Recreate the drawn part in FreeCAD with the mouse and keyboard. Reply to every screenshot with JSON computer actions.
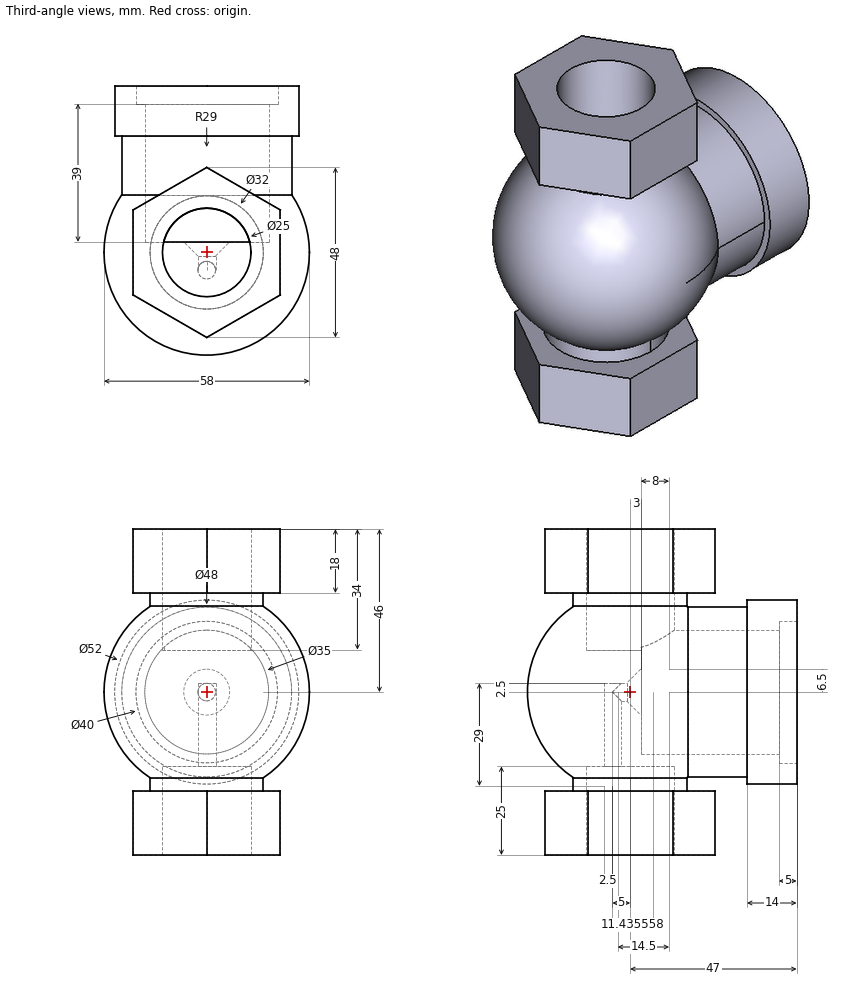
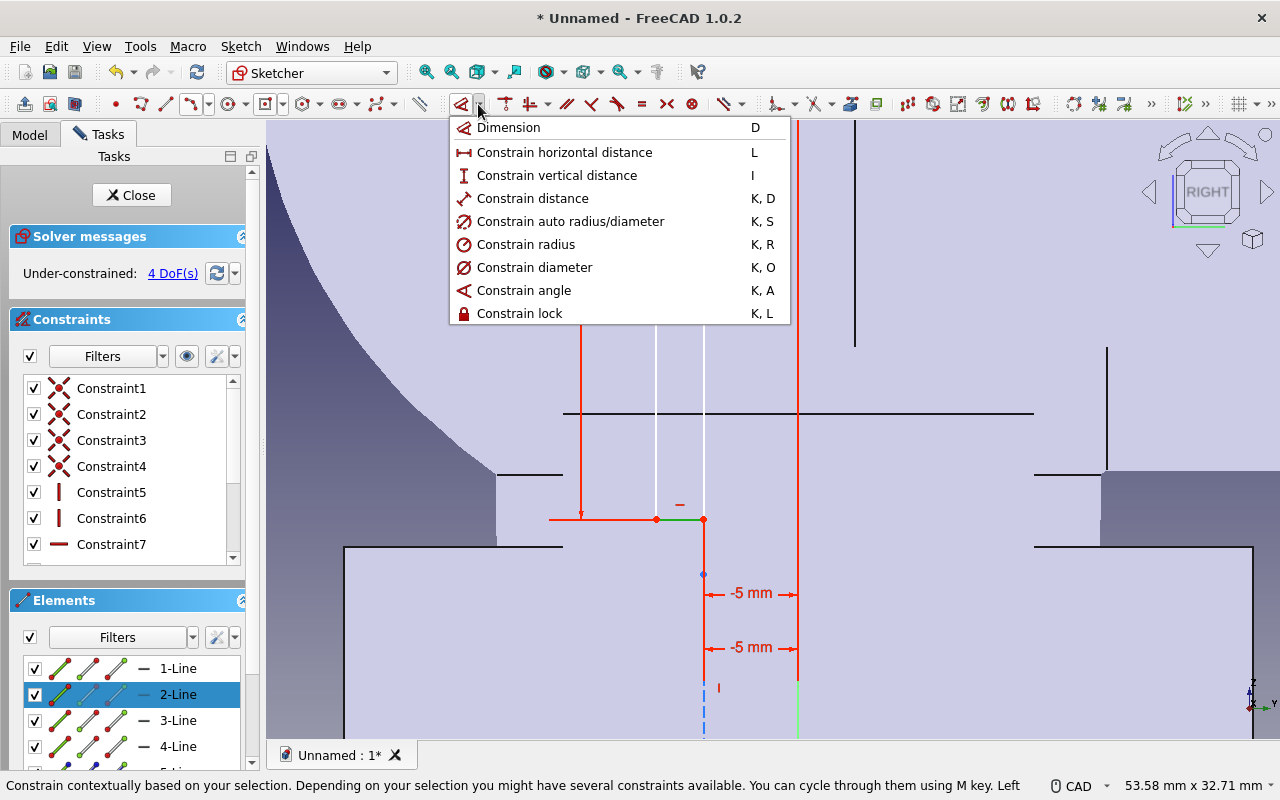
{"action": "left_click", "coordinate": [620, 152]}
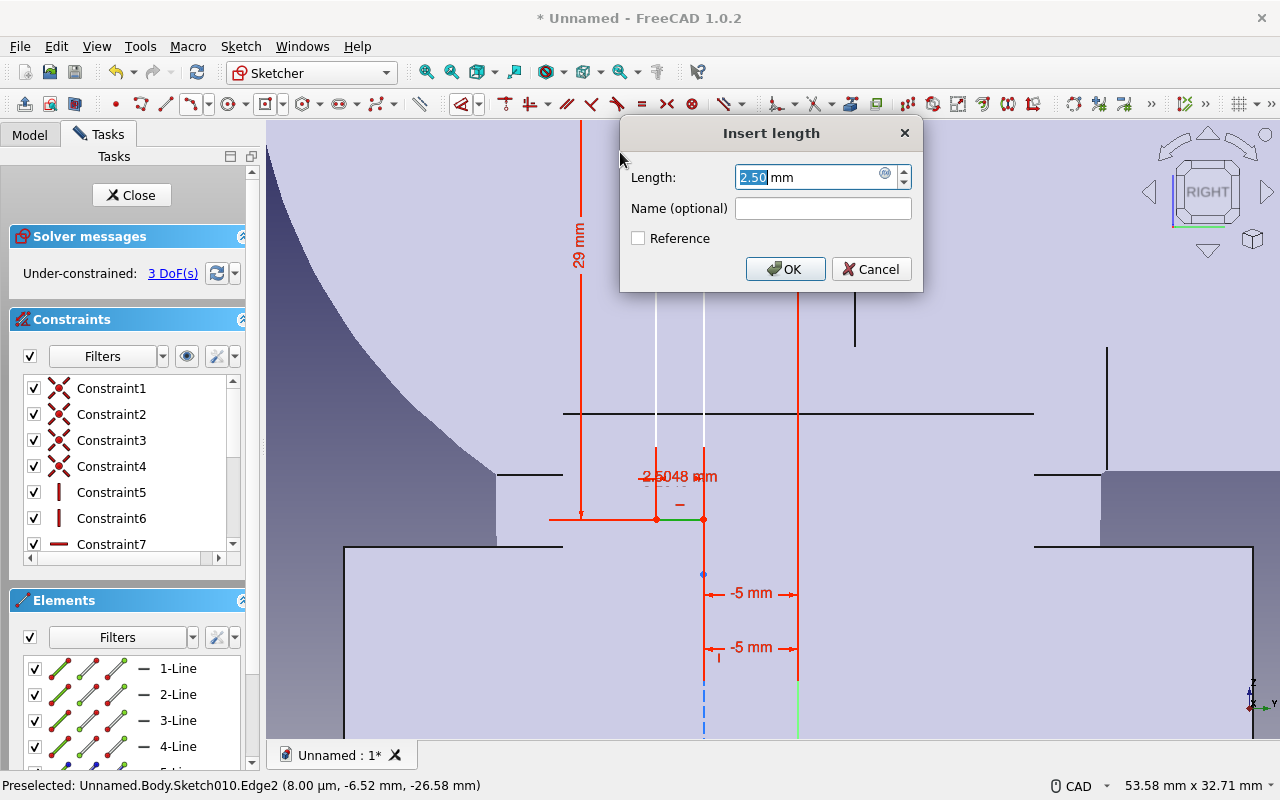
{"action": "type", "text": "2.5"}
{"action": "key", "text": "Return"}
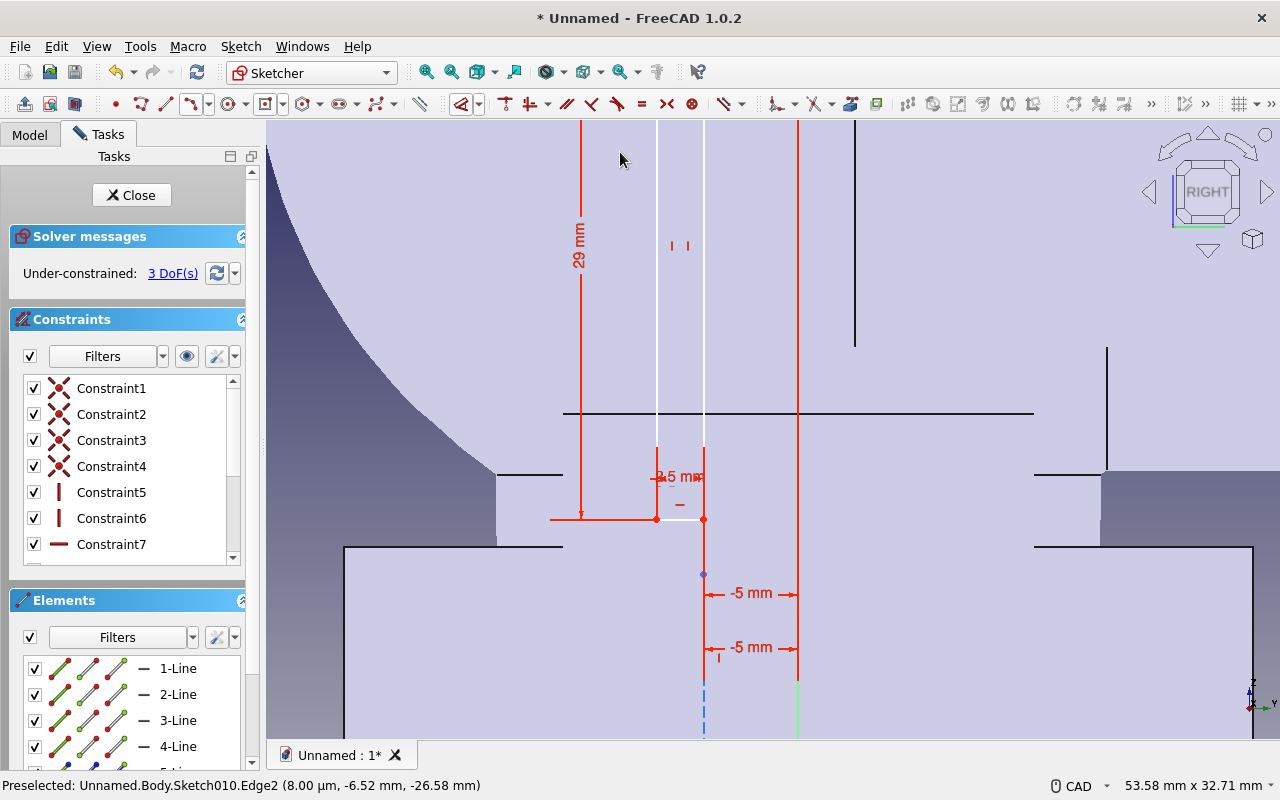
{"action": "scroll", "coordinate": [677, 522], "scroll_direction": "down", "scroll_amount": 3}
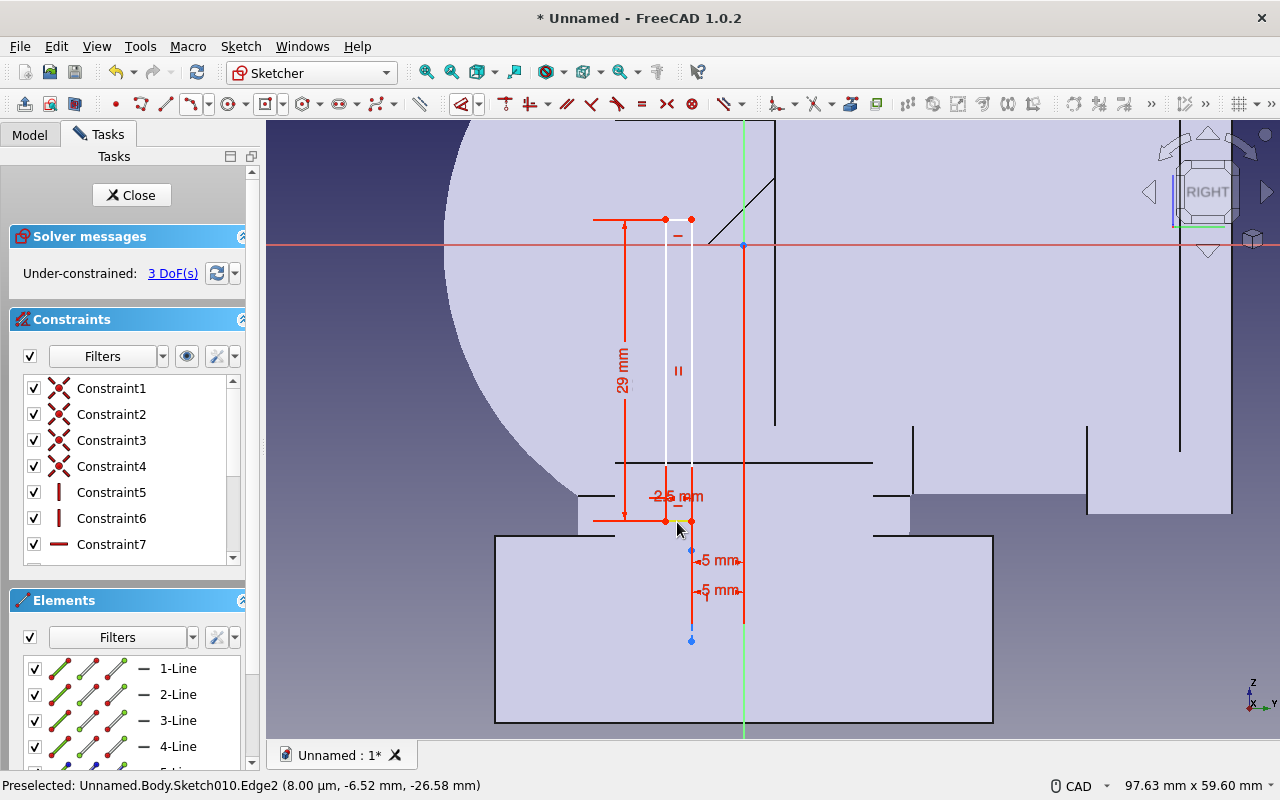
{"action": "scroll", "coordinate": [666, 220], "scroll_direction": "up", "scroll_amount": 3}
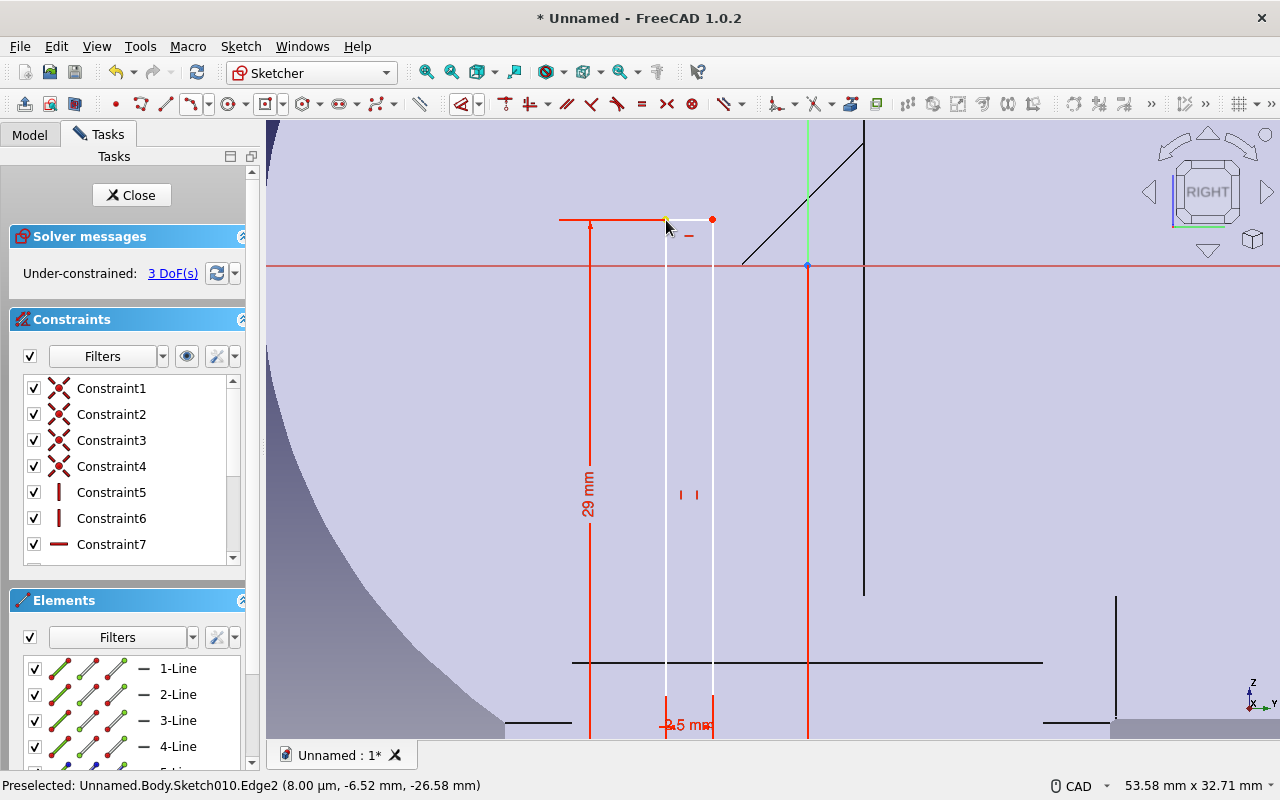
{"action": "left_click", "coordinate": [666, 220]}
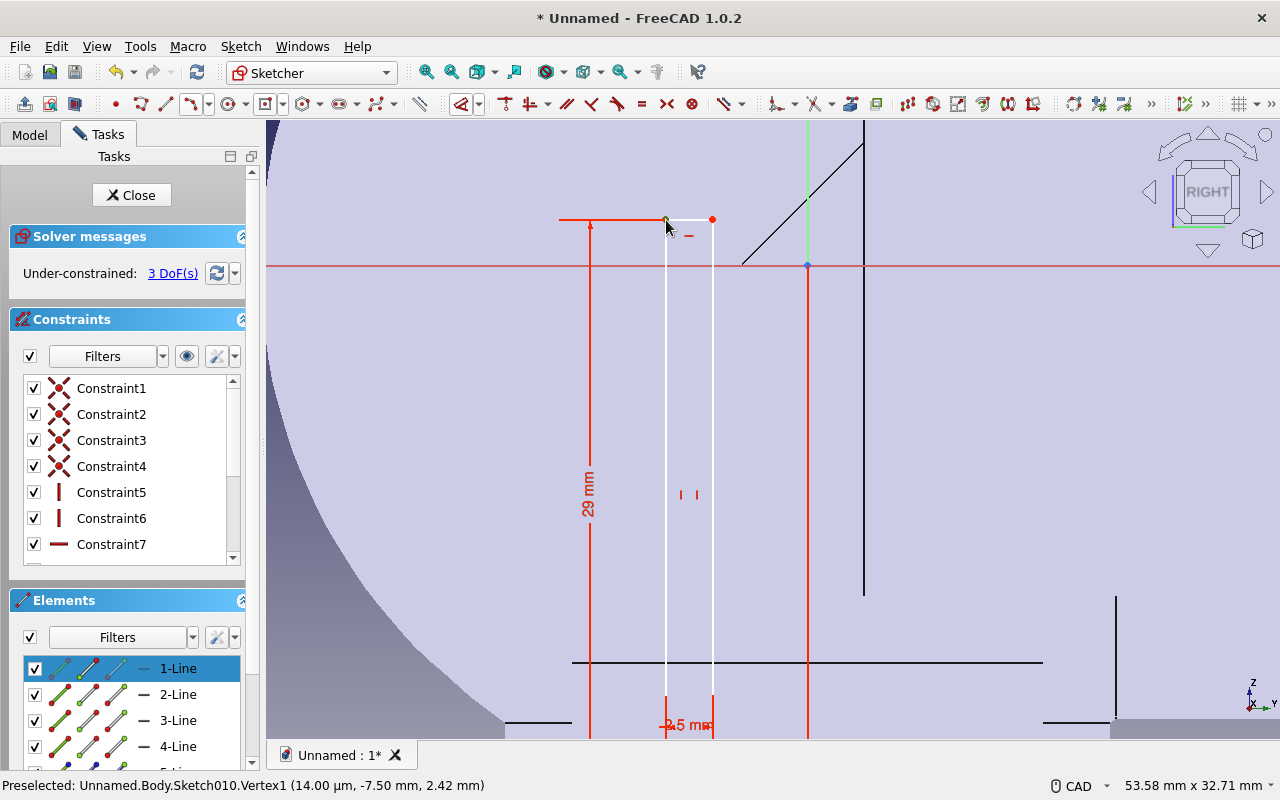
{"action": "key", "text": "i"}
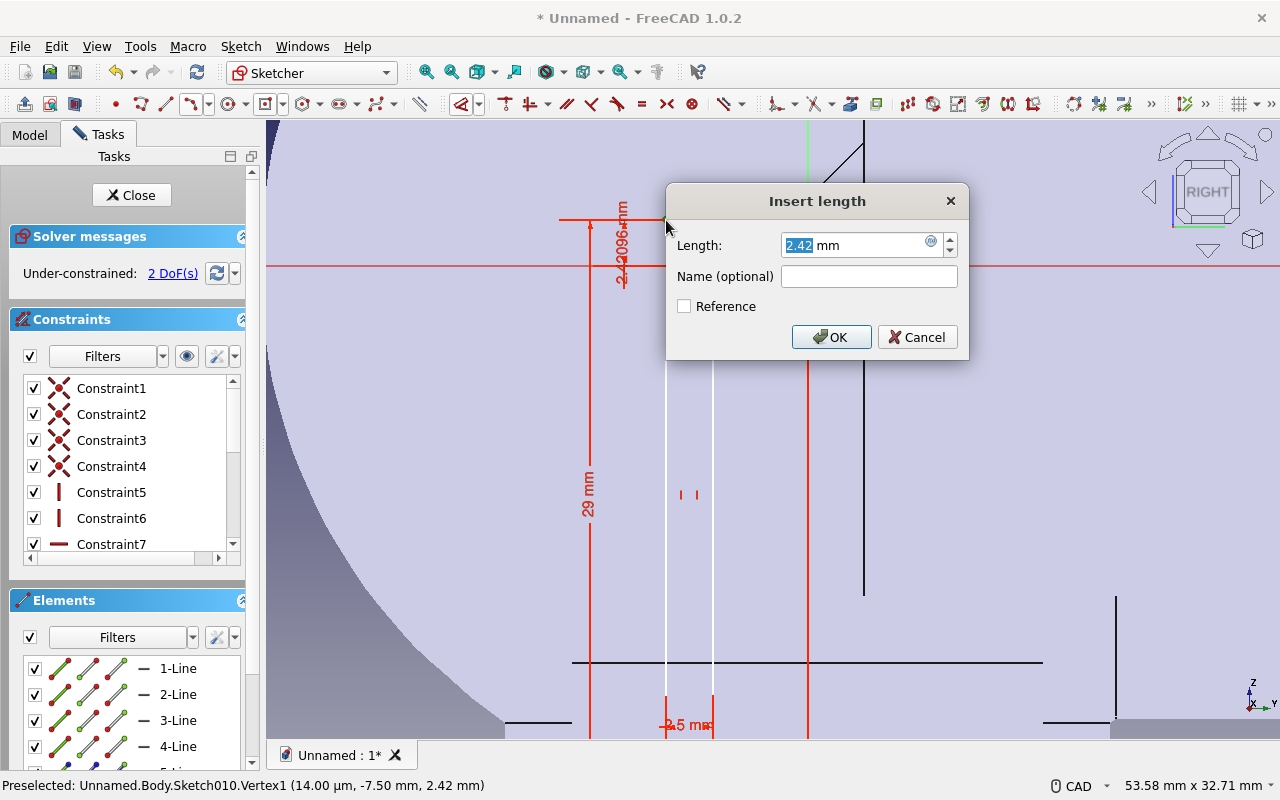
{"action": "type", "text": "2.5"}
{"action": "key", "text": "Return"}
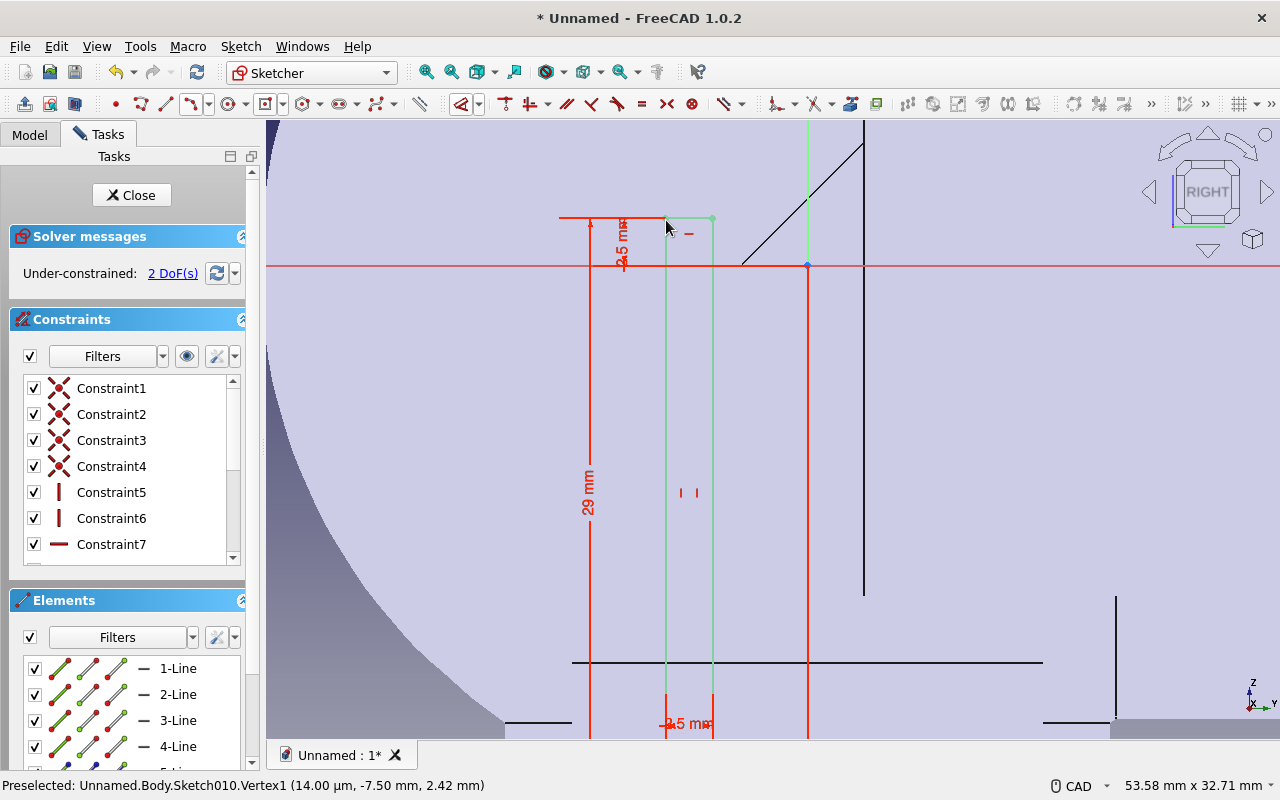
{"action": "left_click", "coordinate": [132, 195]}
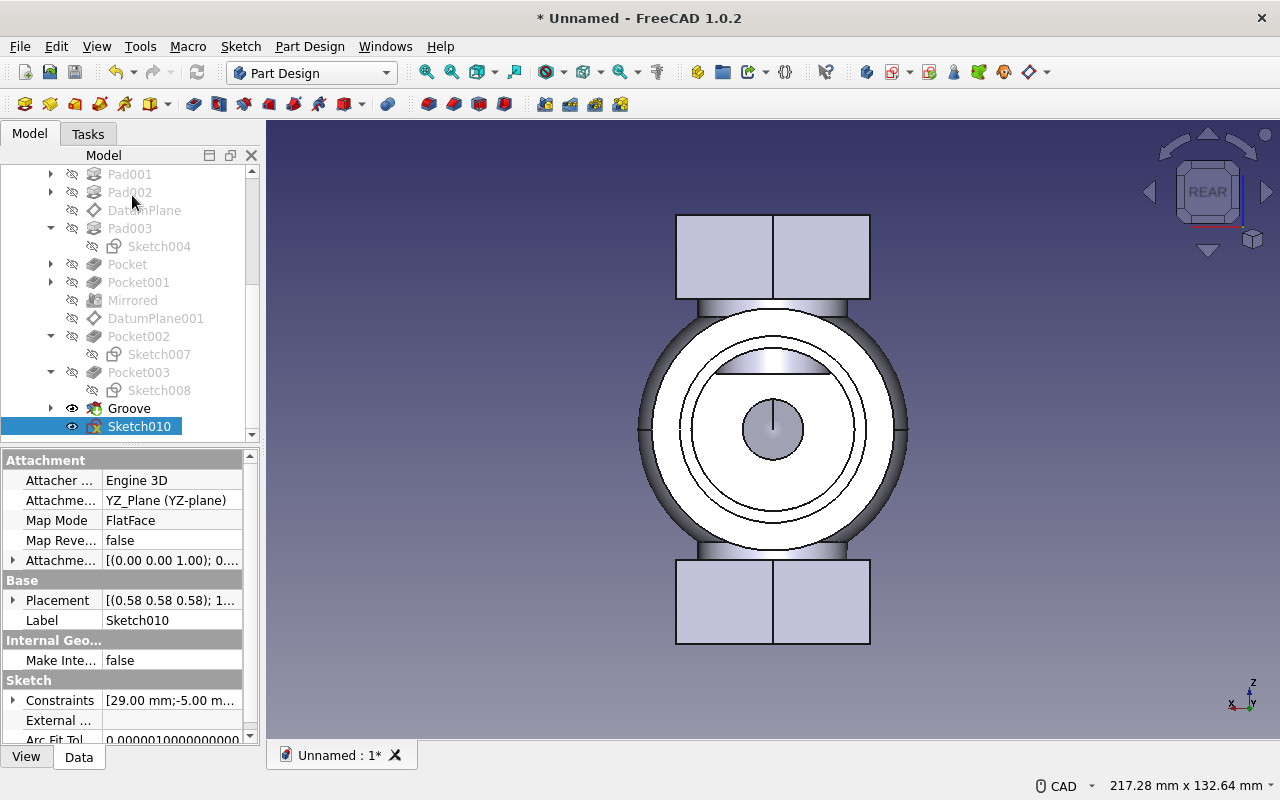
{"action": "left_click", "coordinate": [244, 104]}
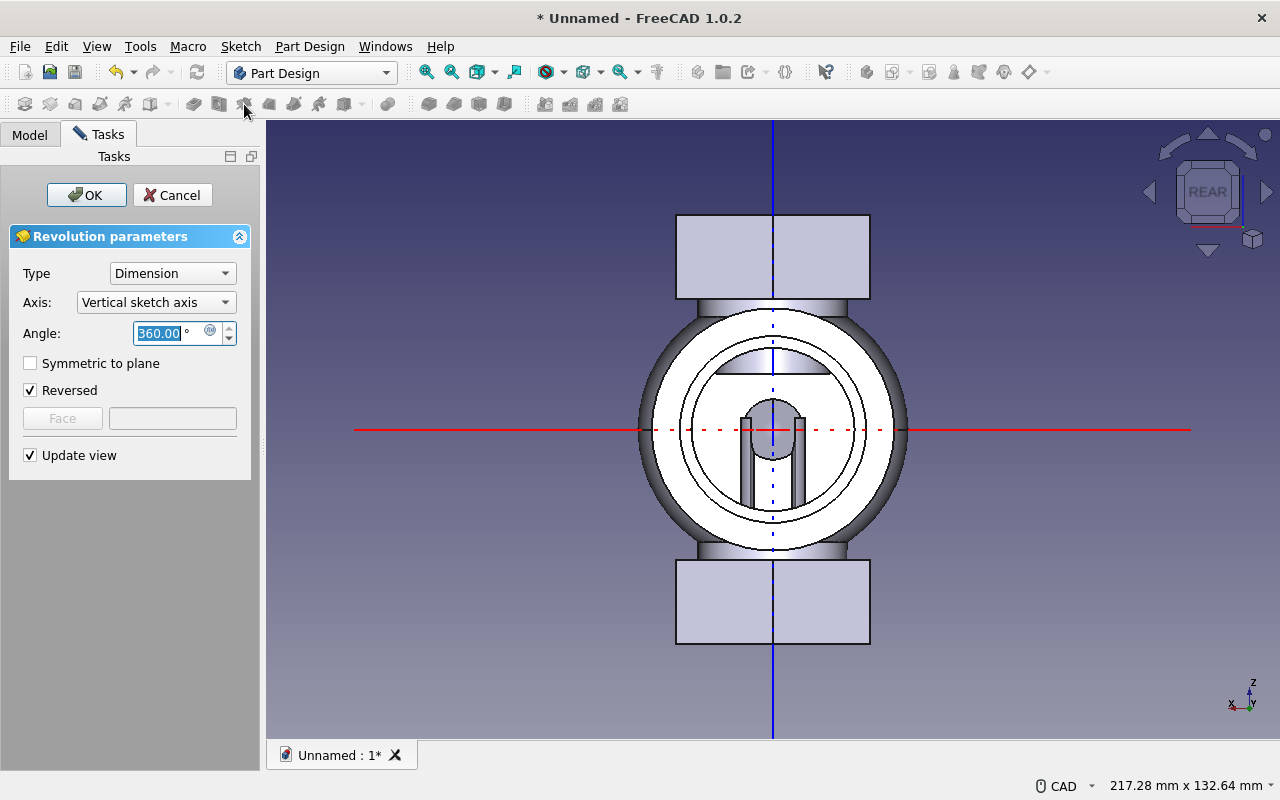
{"action": "left_click", "coordinate": [157, 302]}